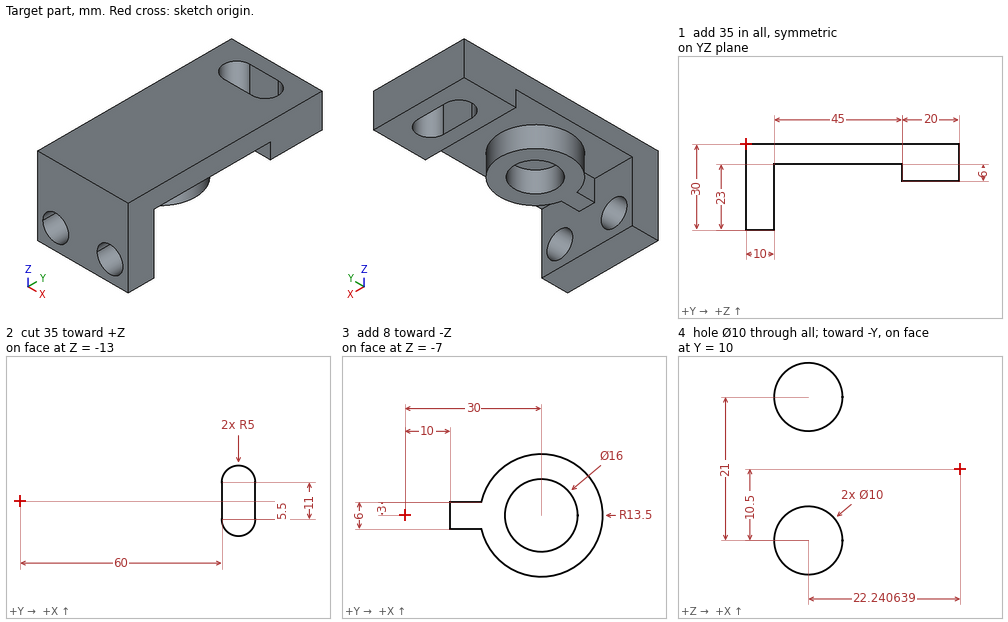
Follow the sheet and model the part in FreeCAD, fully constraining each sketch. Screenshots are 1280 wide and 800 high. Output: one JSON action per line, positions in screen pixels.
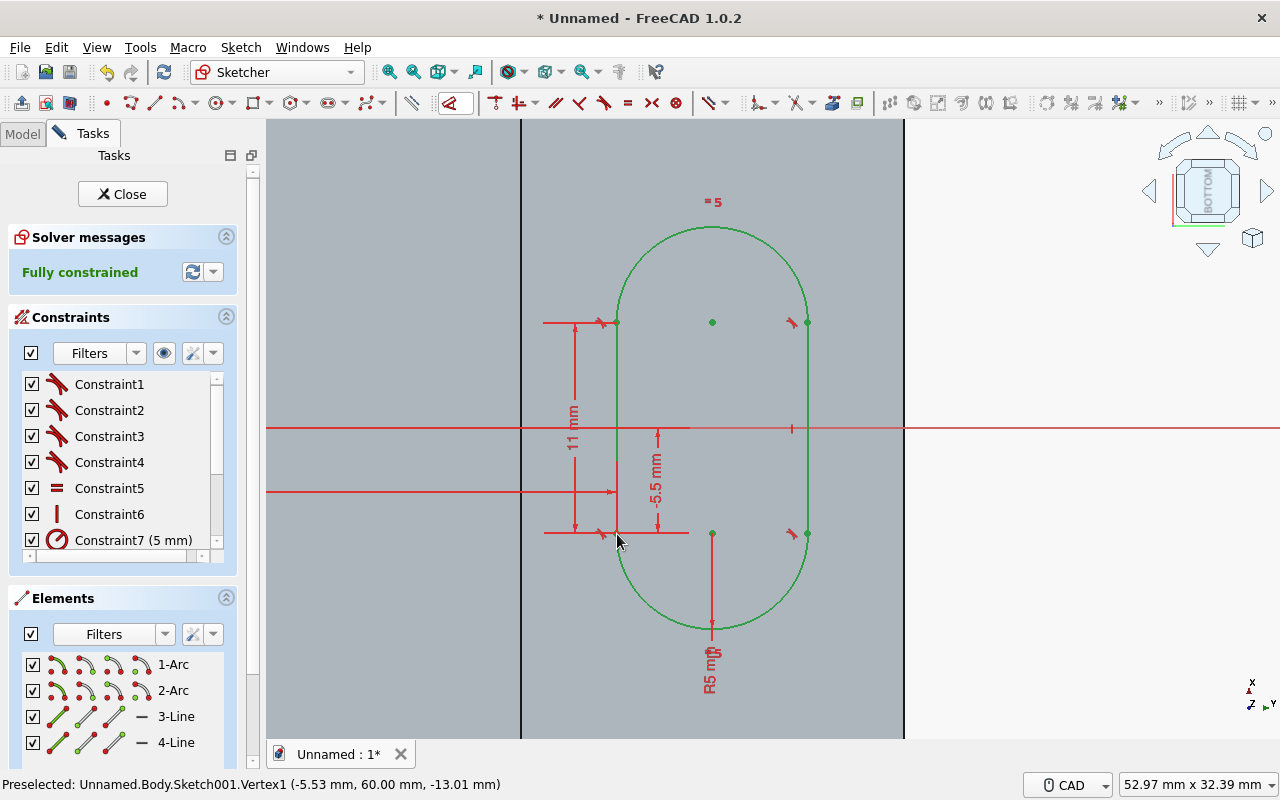
{"action": "left_click", "coordinate": [123, 194]}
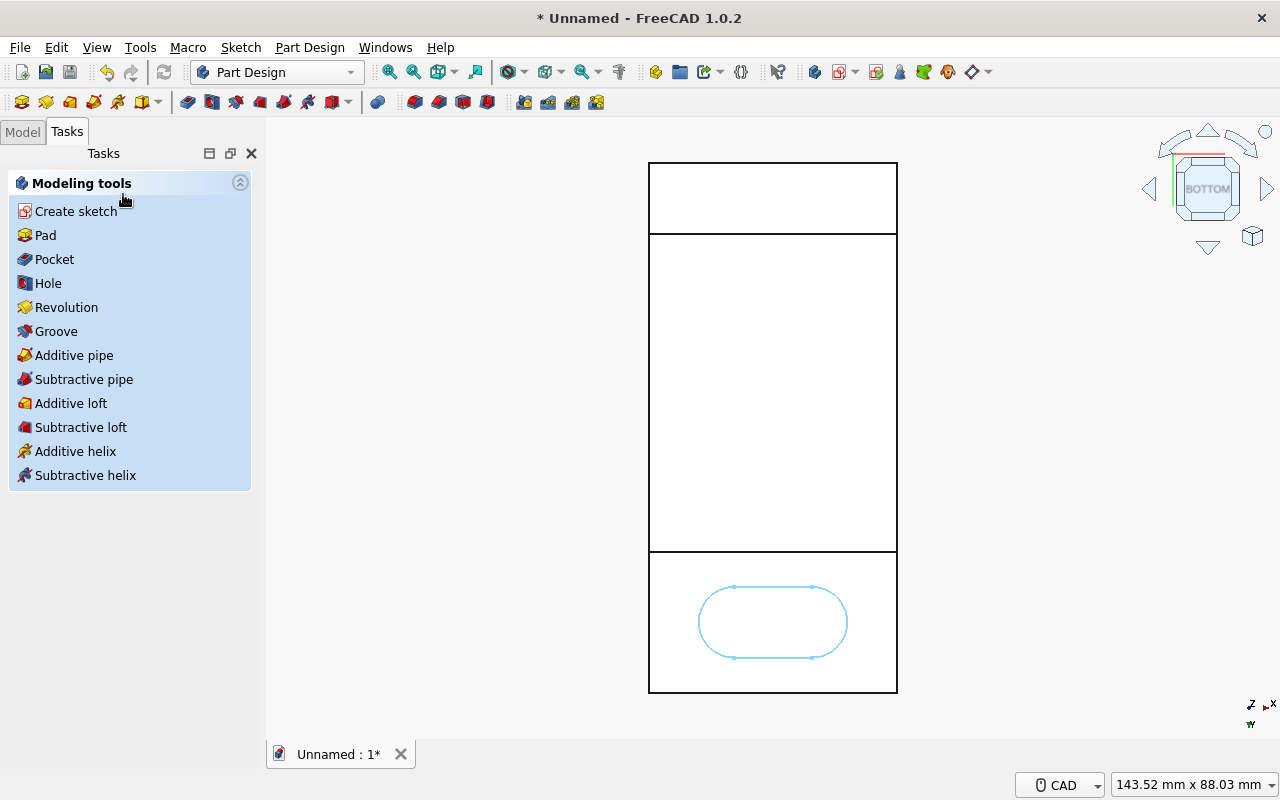
{"action": "left_click", "coordinate": [188, 102]}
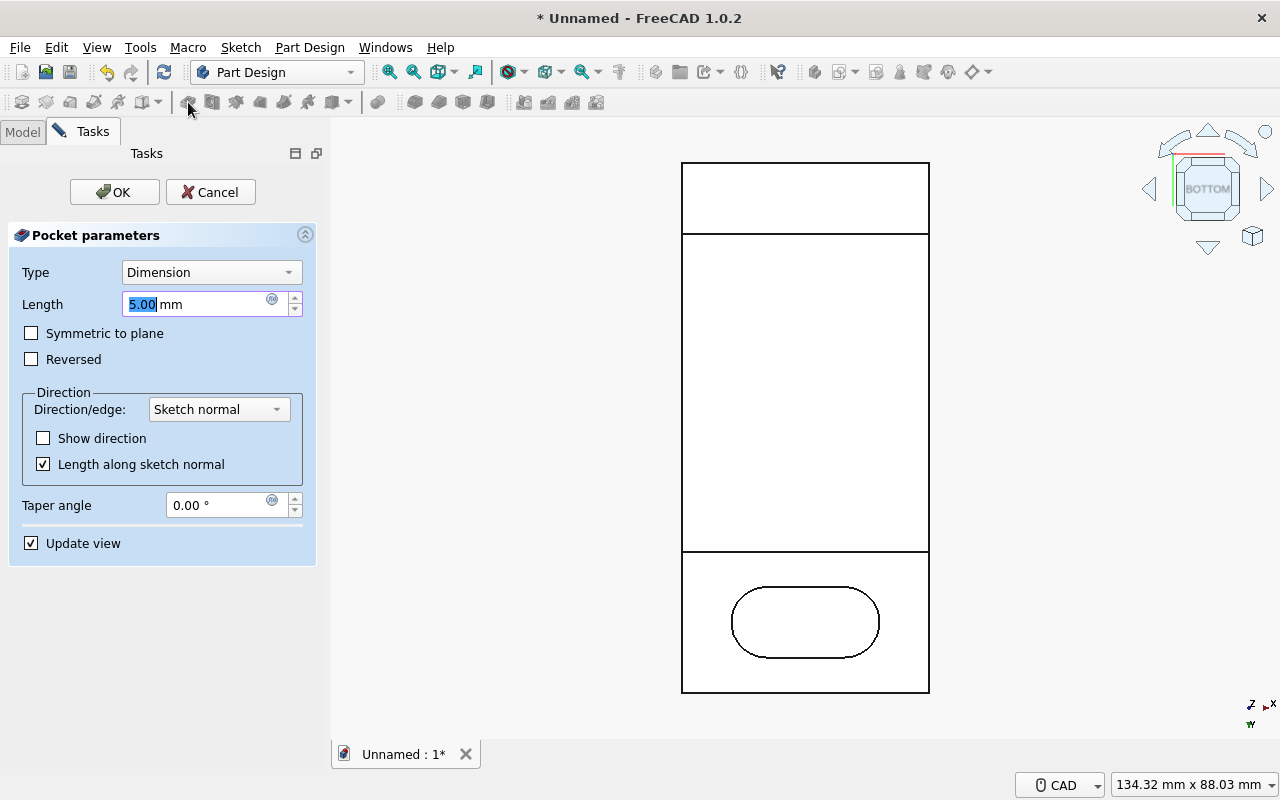
{"action": "type", "text": "35"}
{"action": "key", "text": "Tab"}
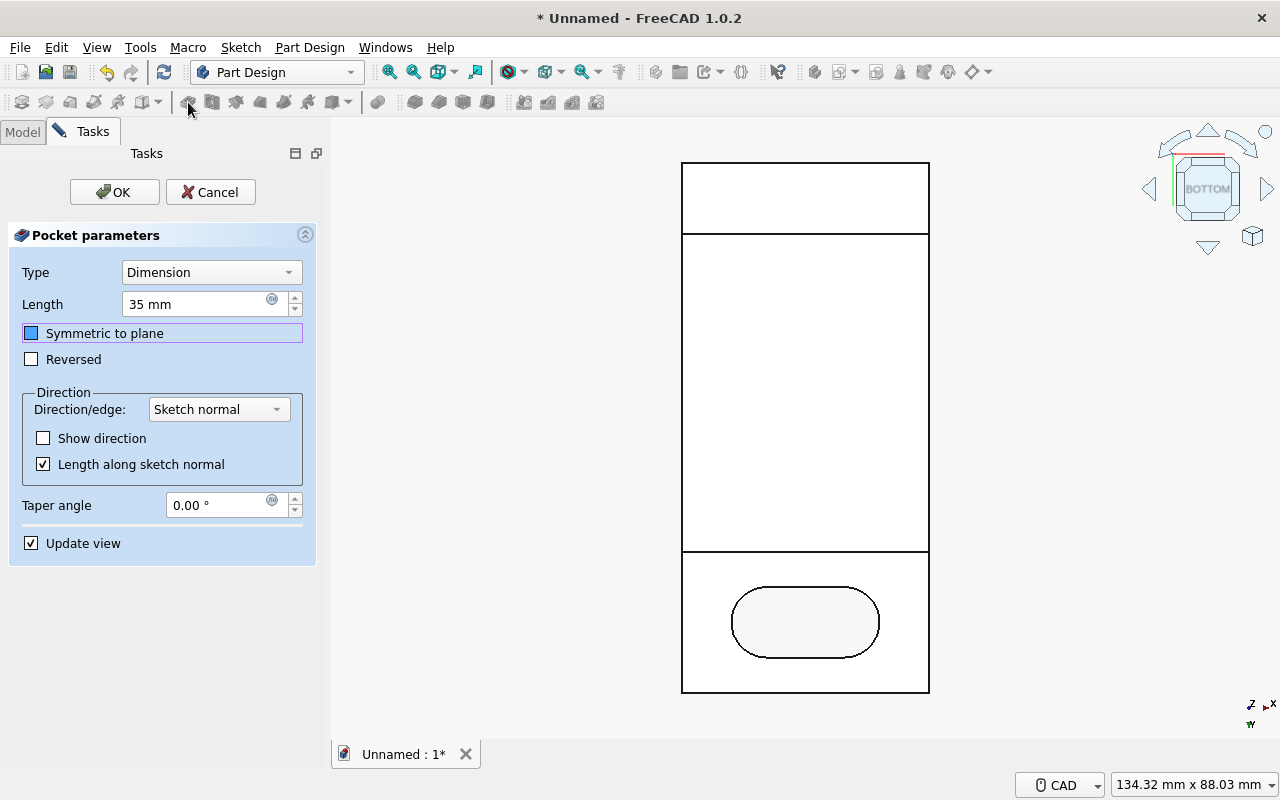
{"action": "left_click", "coordinate": [115, 192]}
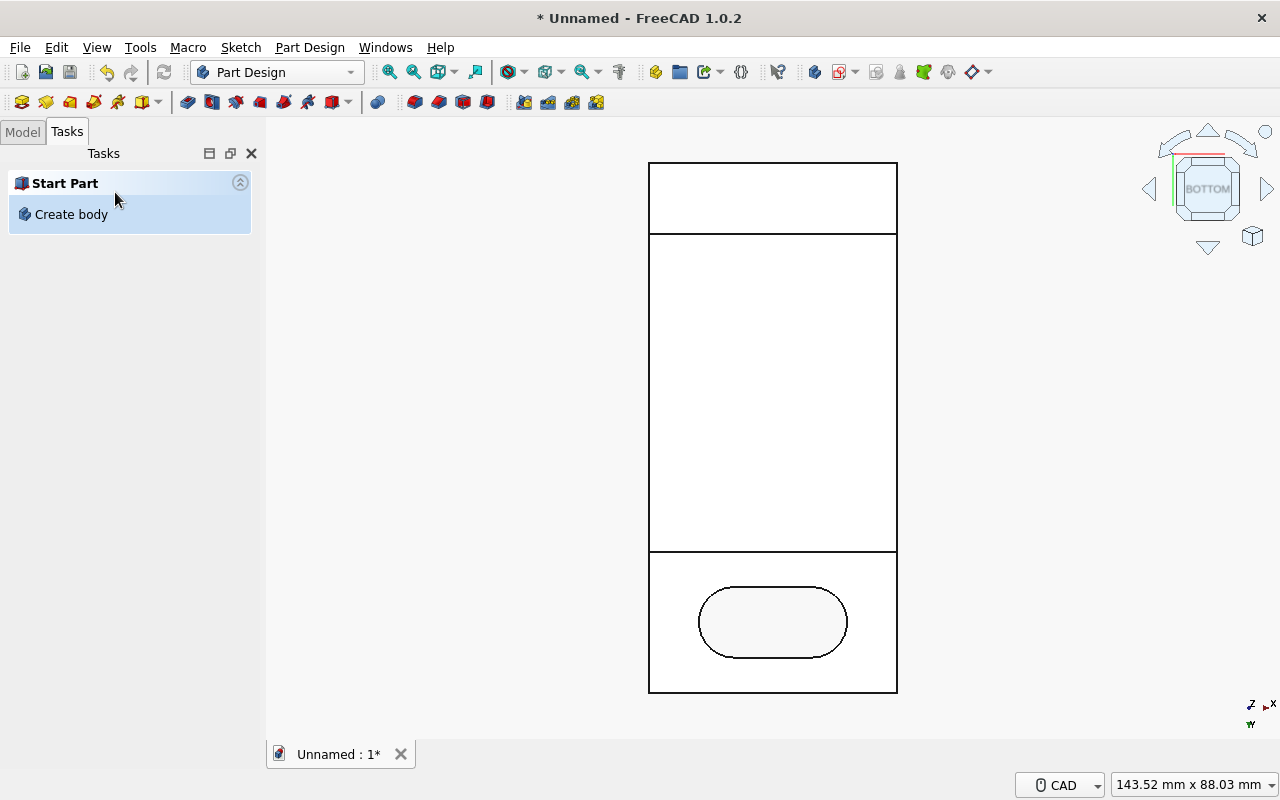
{"action": "left_click", "coordinate": [773, 392]}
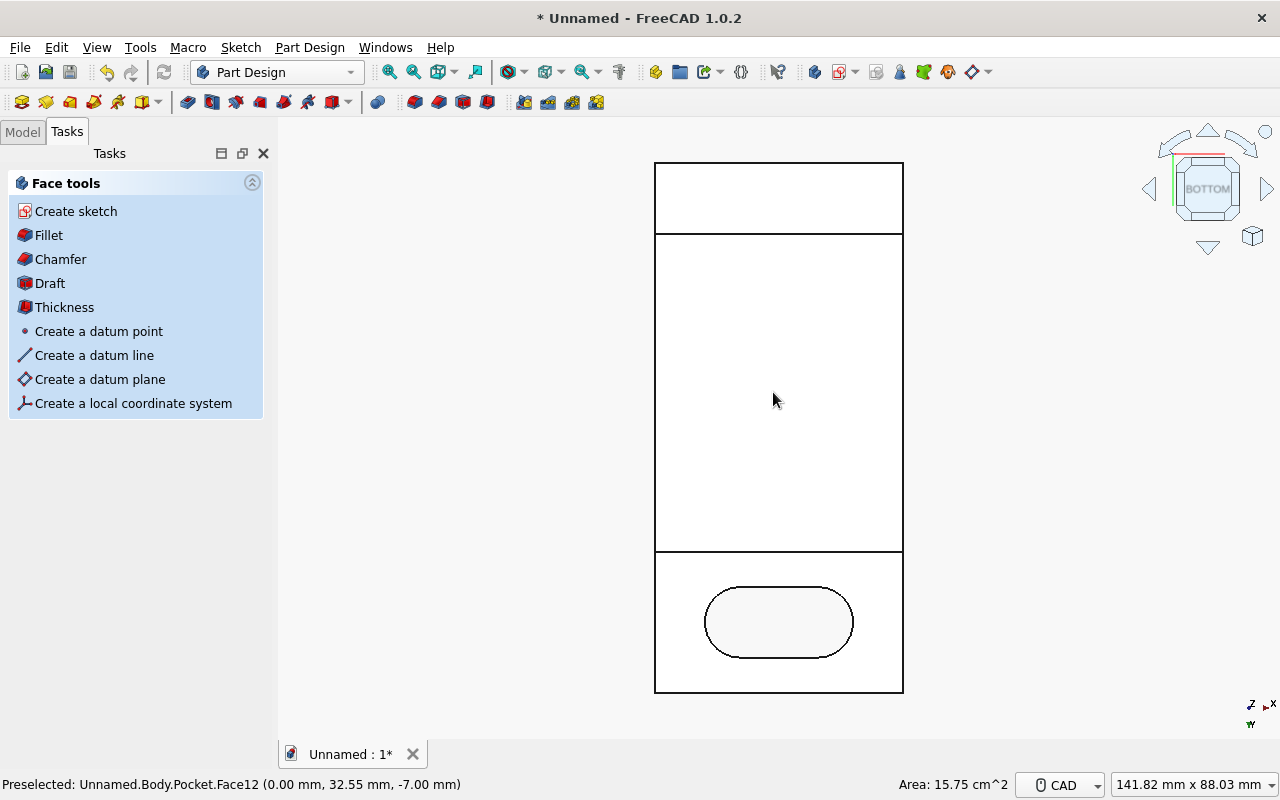
{"action": "left_click", "coordinate": [840, 72]}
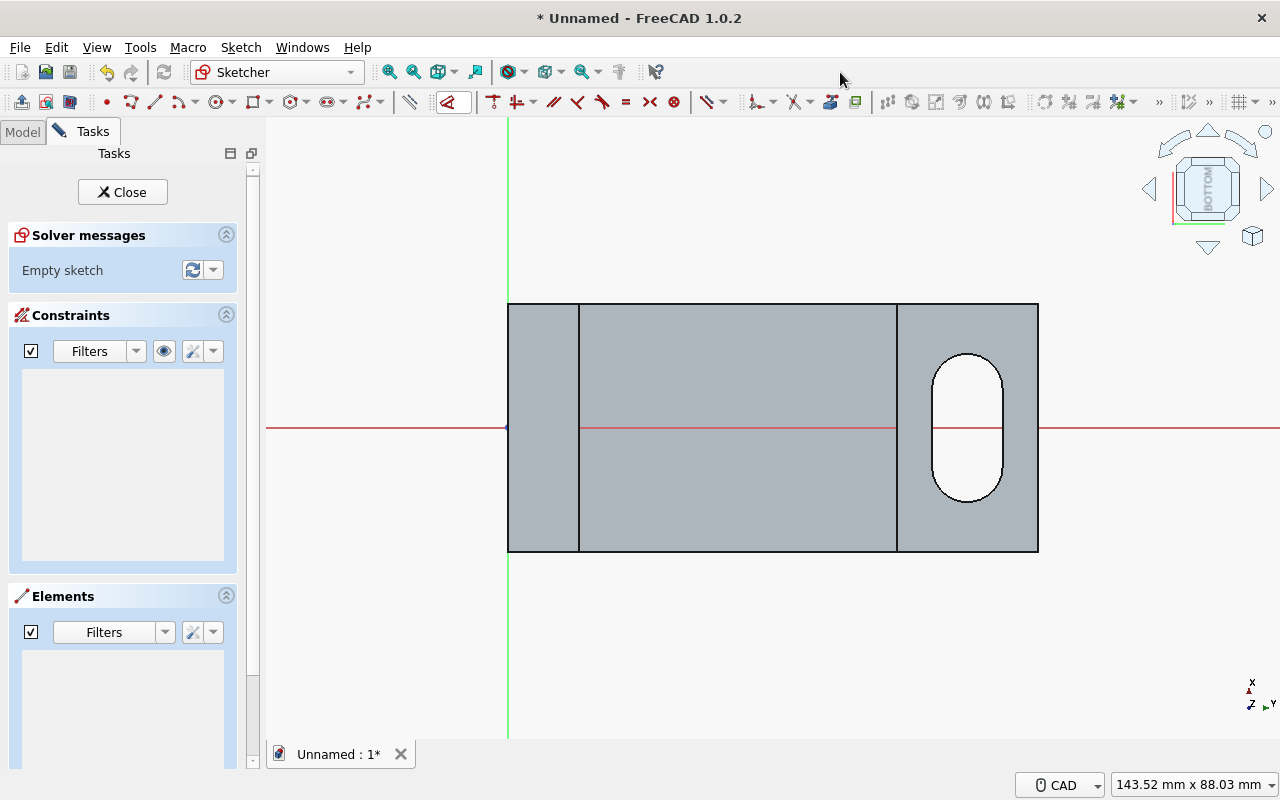
{"action": "scroll", "coordinate": [610, 428], "scroll_direction": "up", "scroll_amount": 3}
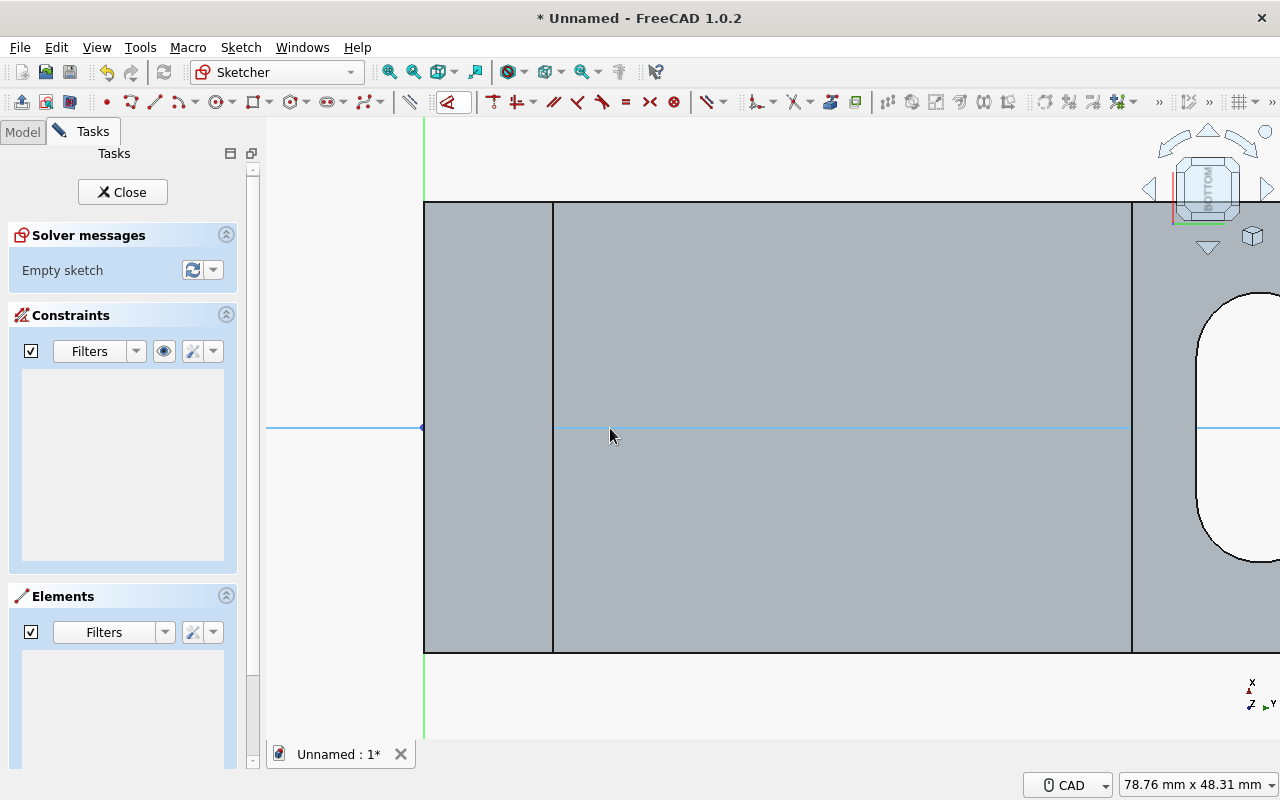
{"action": "key", "text": "g m"}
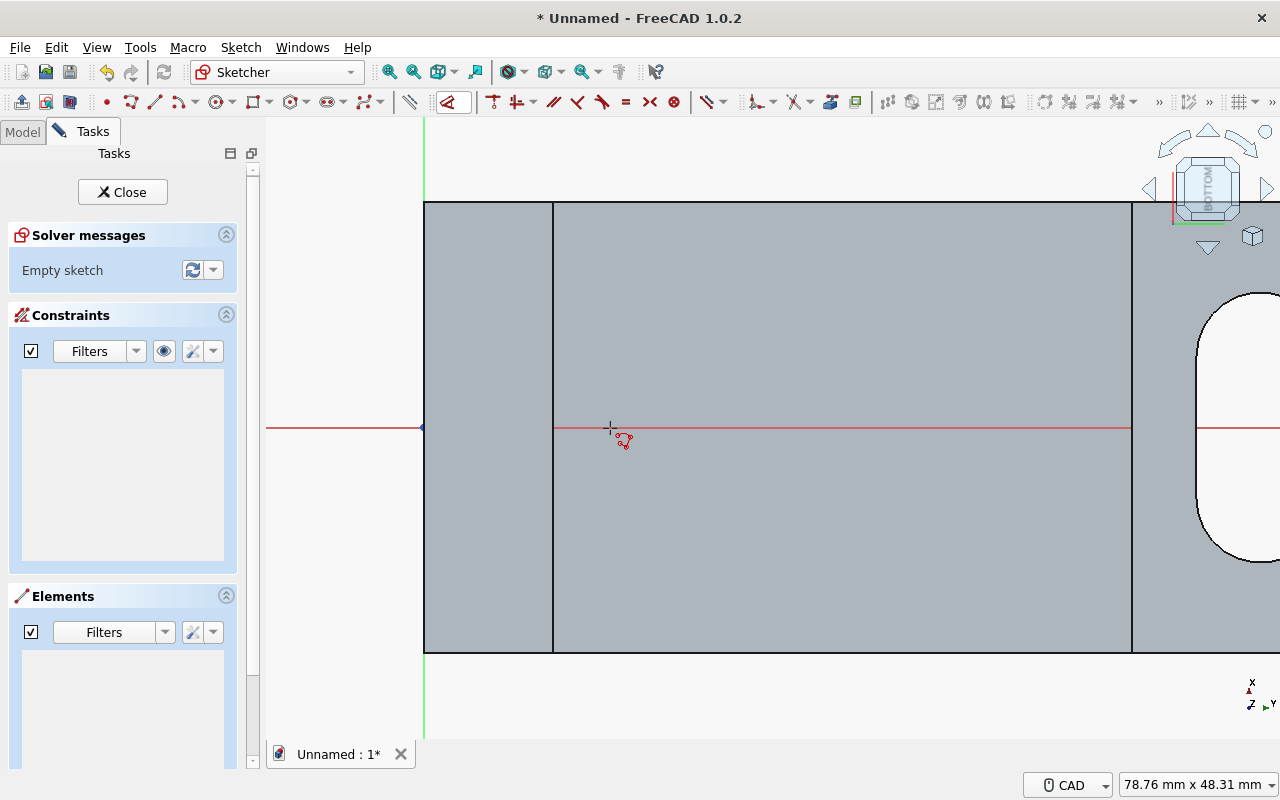
{"action": "left_click", "coordinate": [641, 389]}
{"action": "left_click", "coordinate": [553, 389]}
{"action": "left_click", "coordinate": [553, 466]}
{"action": "left_click", "coordinate": [641, 466]}
{"action": "right_click", "coordinate": [641, 466]}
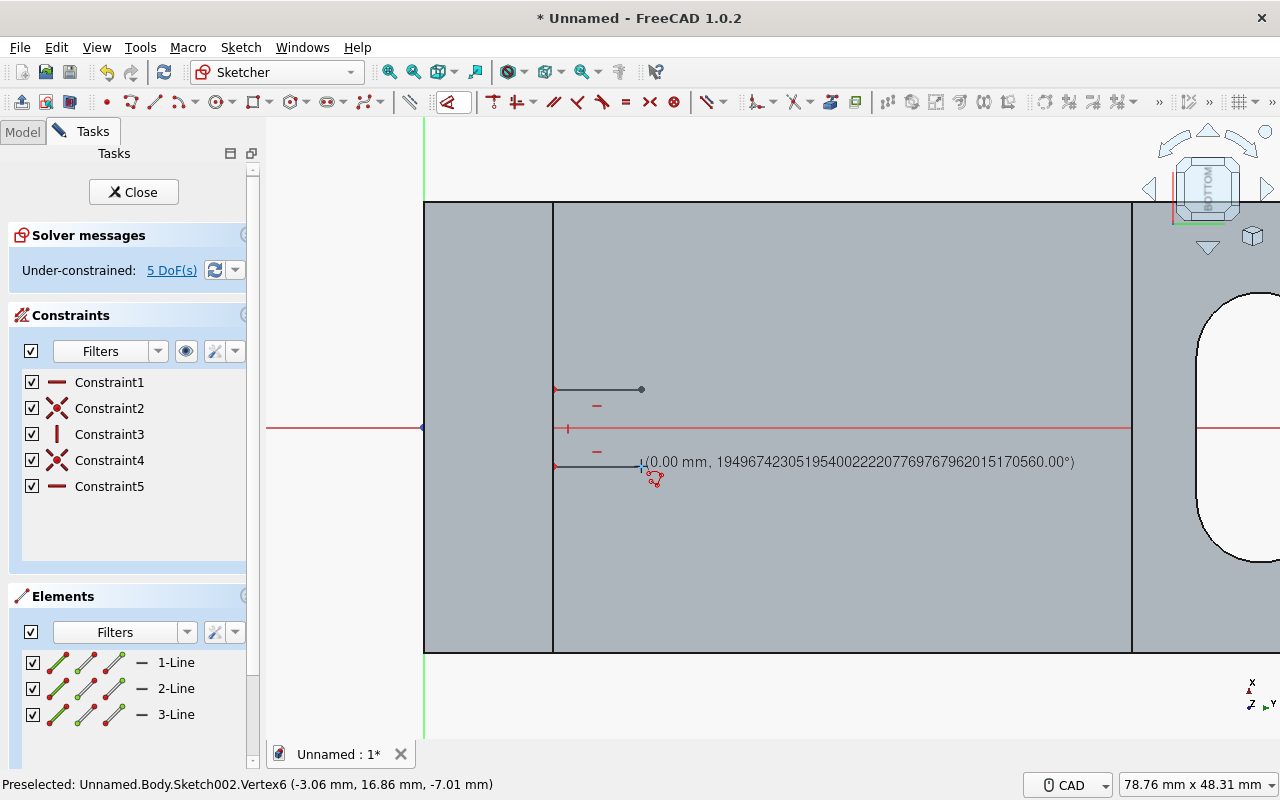
{"action": "left_click", "coordinate": [198, 102]}